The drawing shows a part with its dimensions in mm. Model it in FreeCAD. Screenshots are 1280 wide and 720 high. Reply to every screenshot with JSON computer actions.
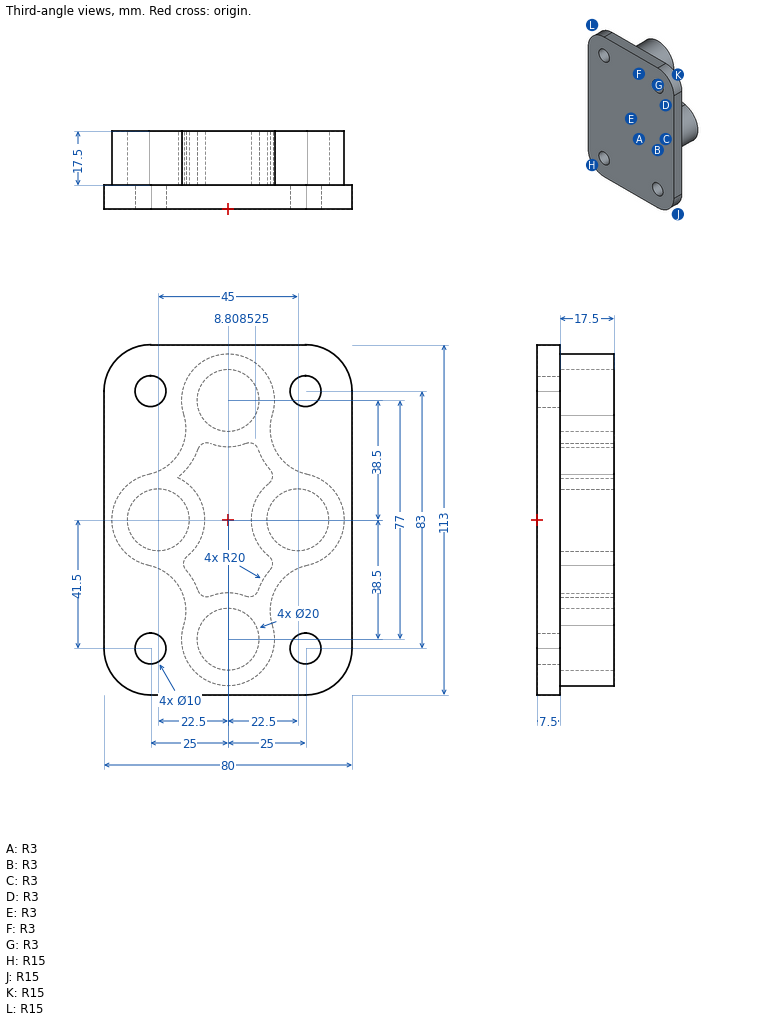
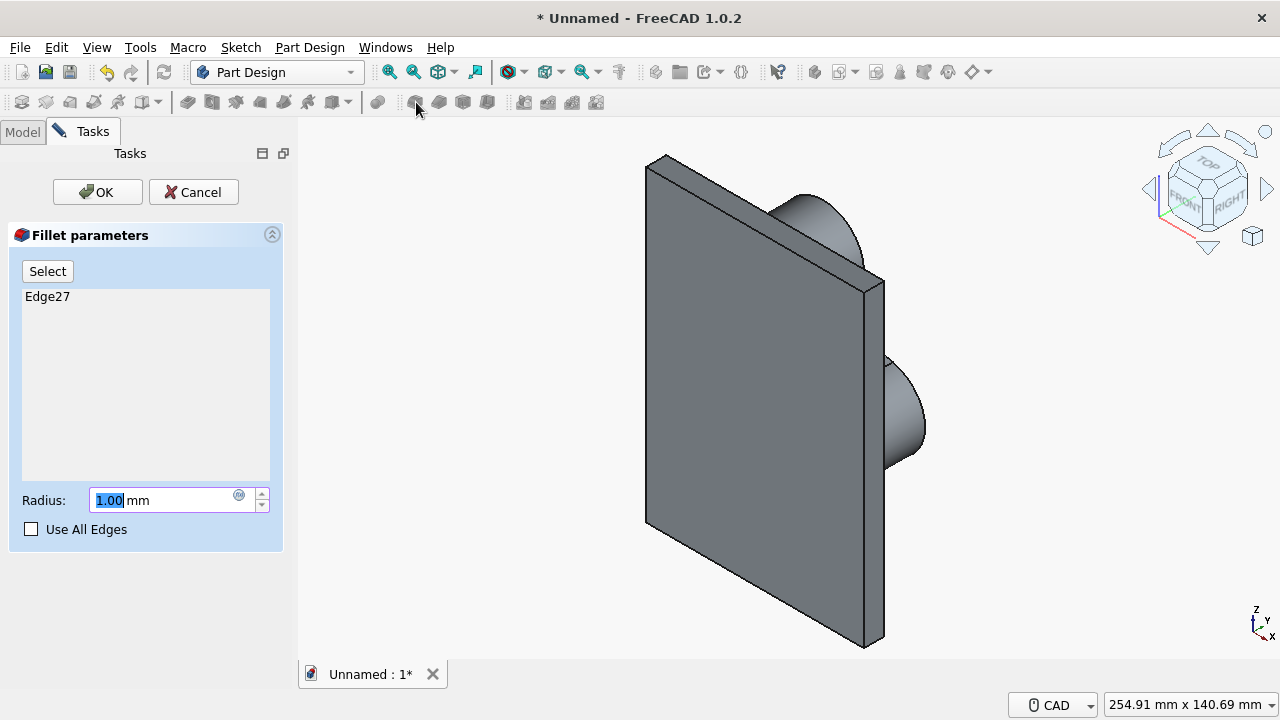
{"action": "type", "text": "3"}
{"action": "key", "text": "Tab"}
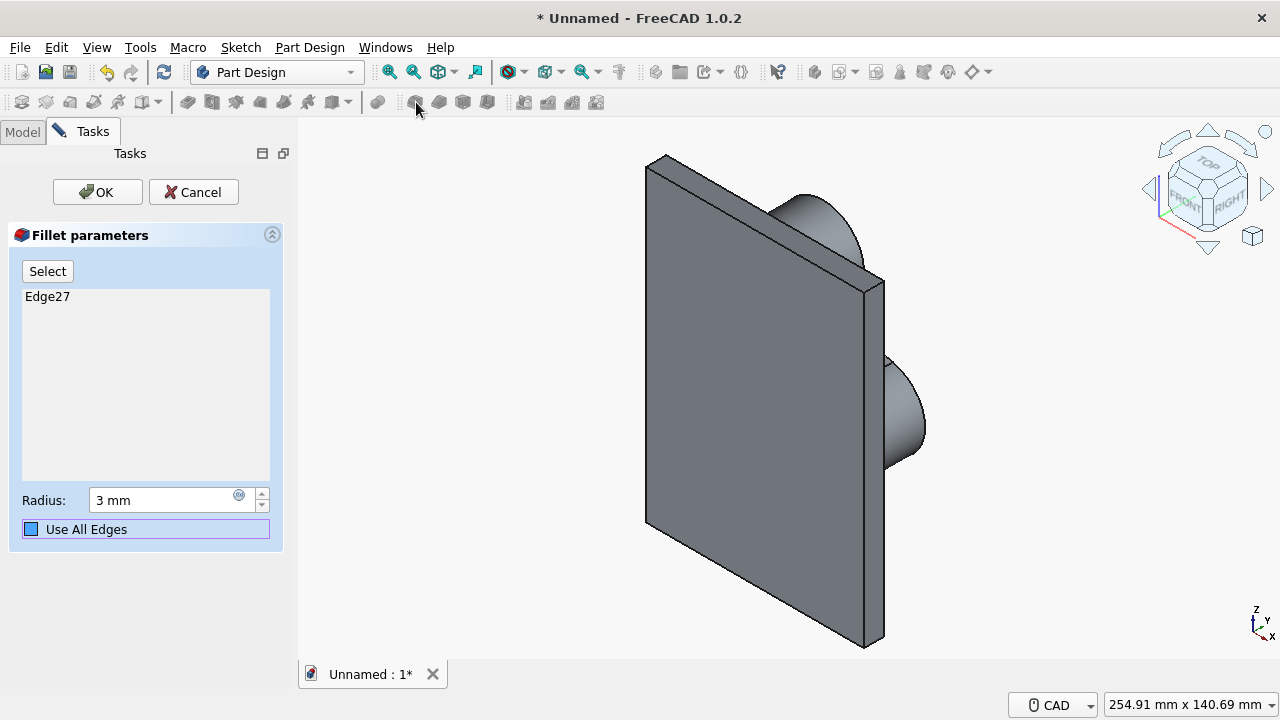
{"action": "left_click", "coordinate": [98, 192]}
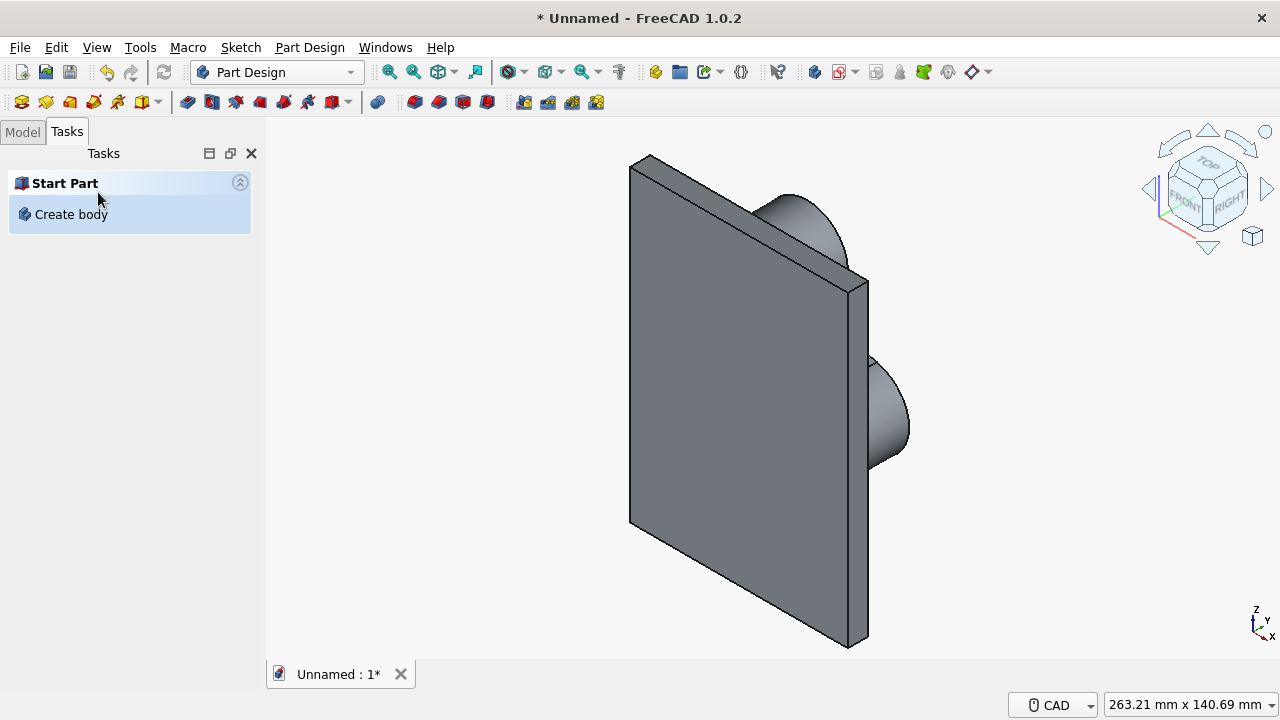
{"action": "key", "text": "2"}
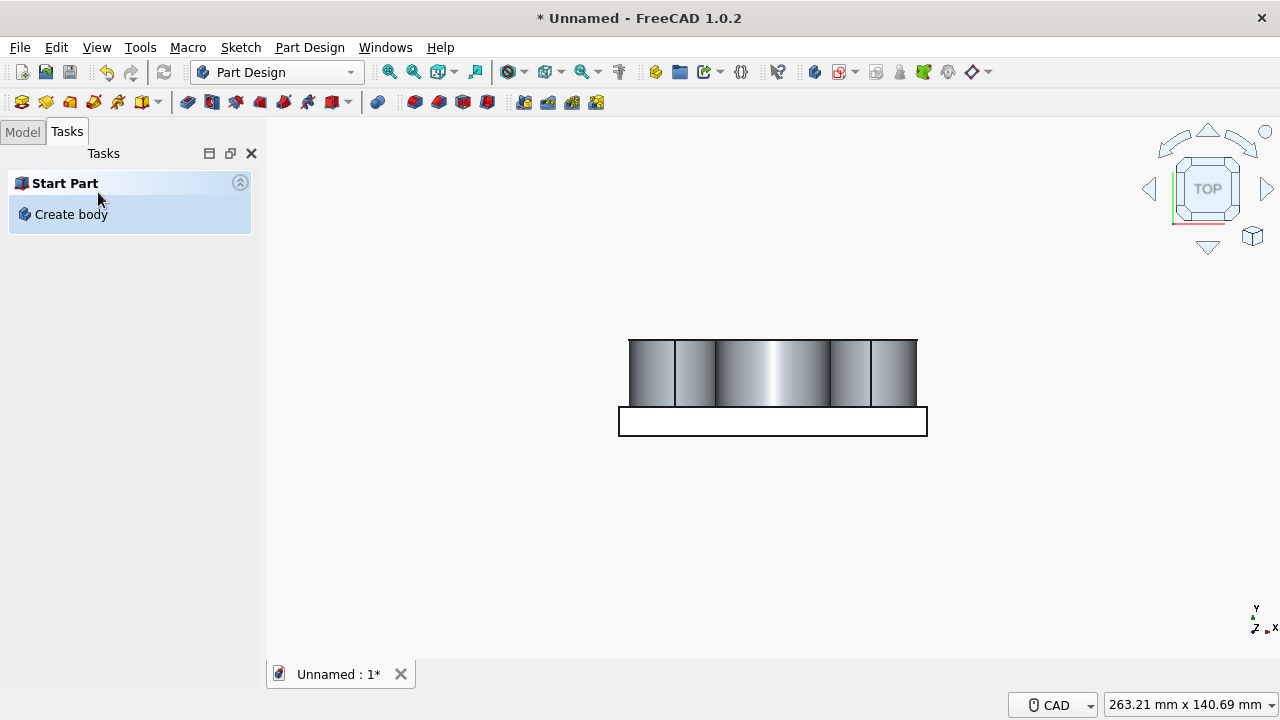
{"action": "left_click", "coordinate": [390, 72]}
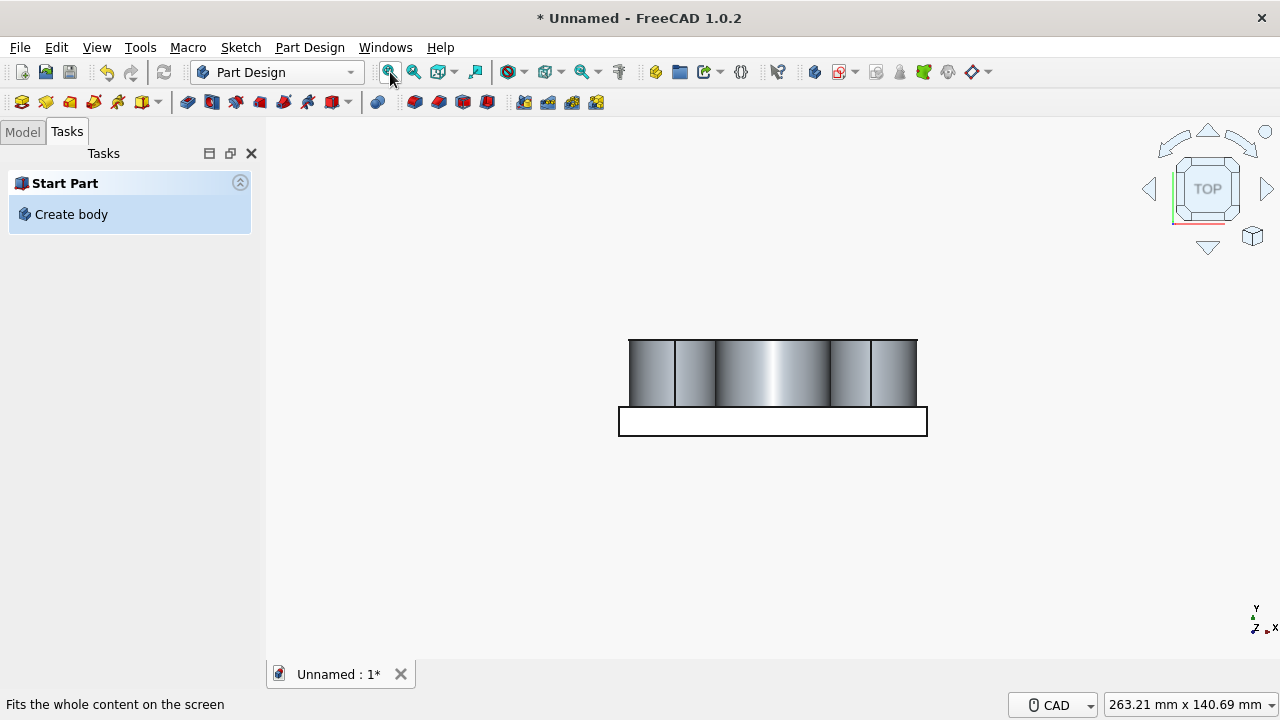
{"action": "key", "text": "0"}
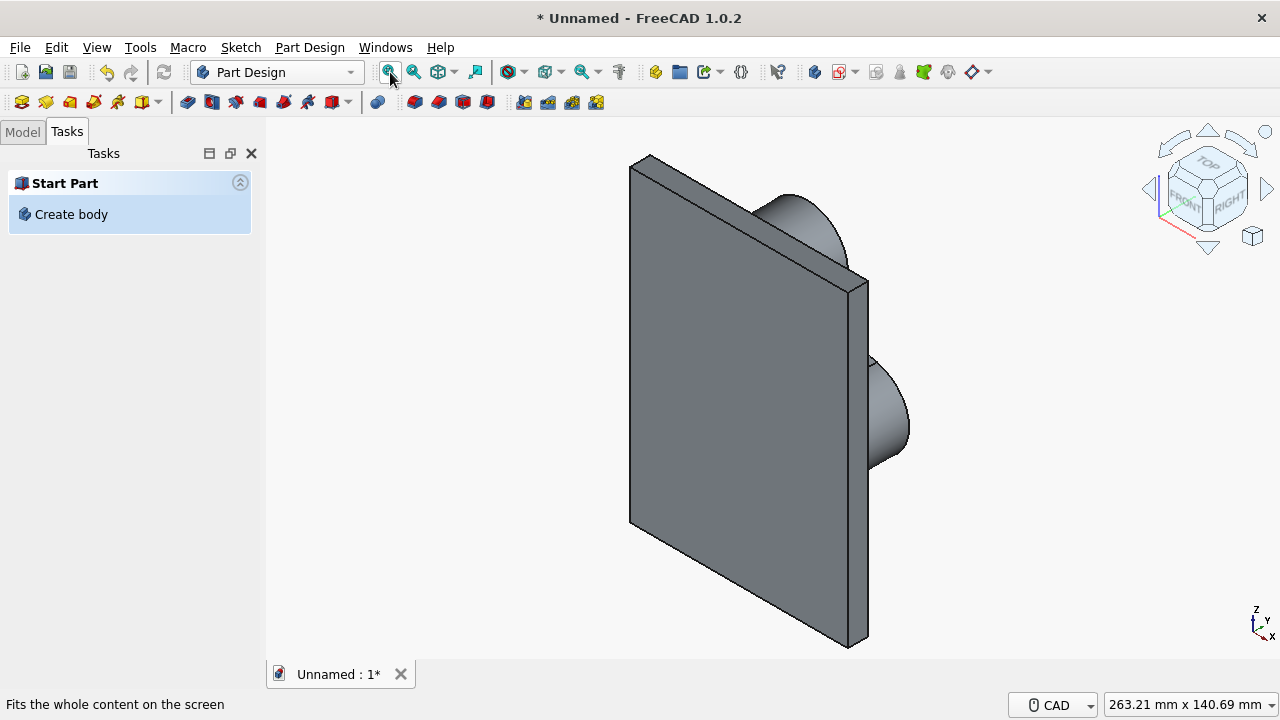
{"action": "key", "text": "1"}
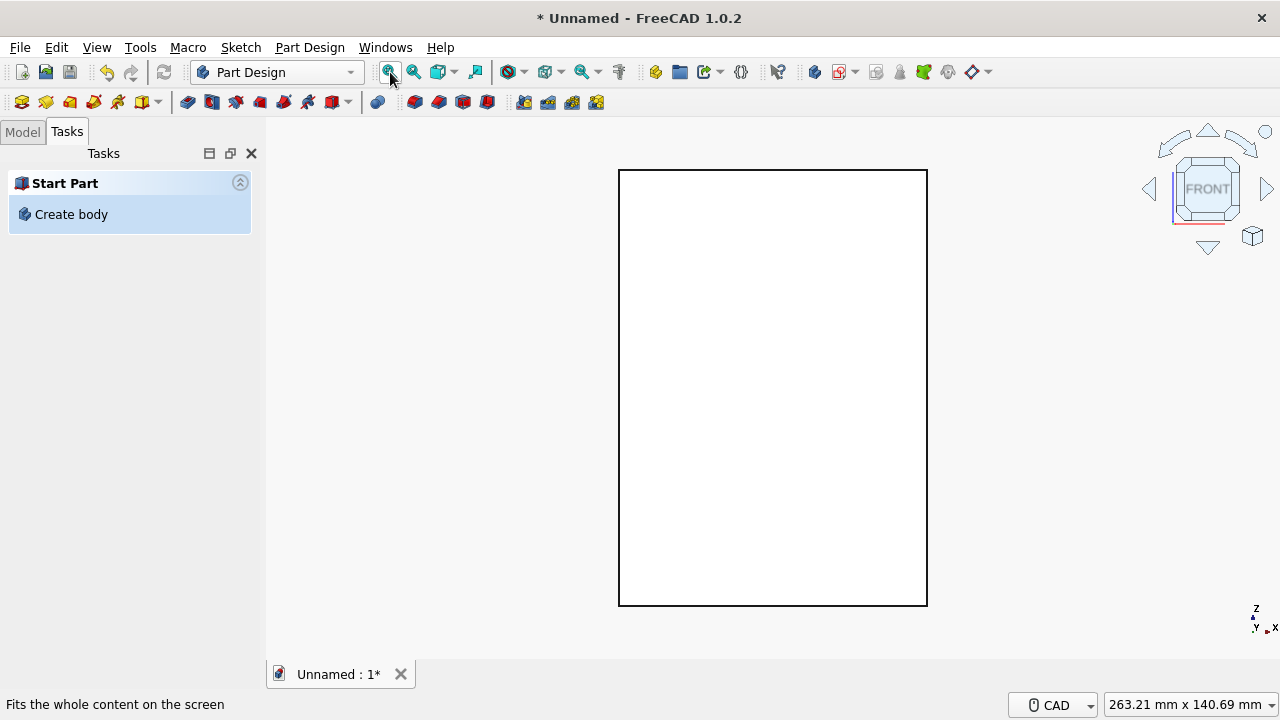
{"action": "key", "text": "3"}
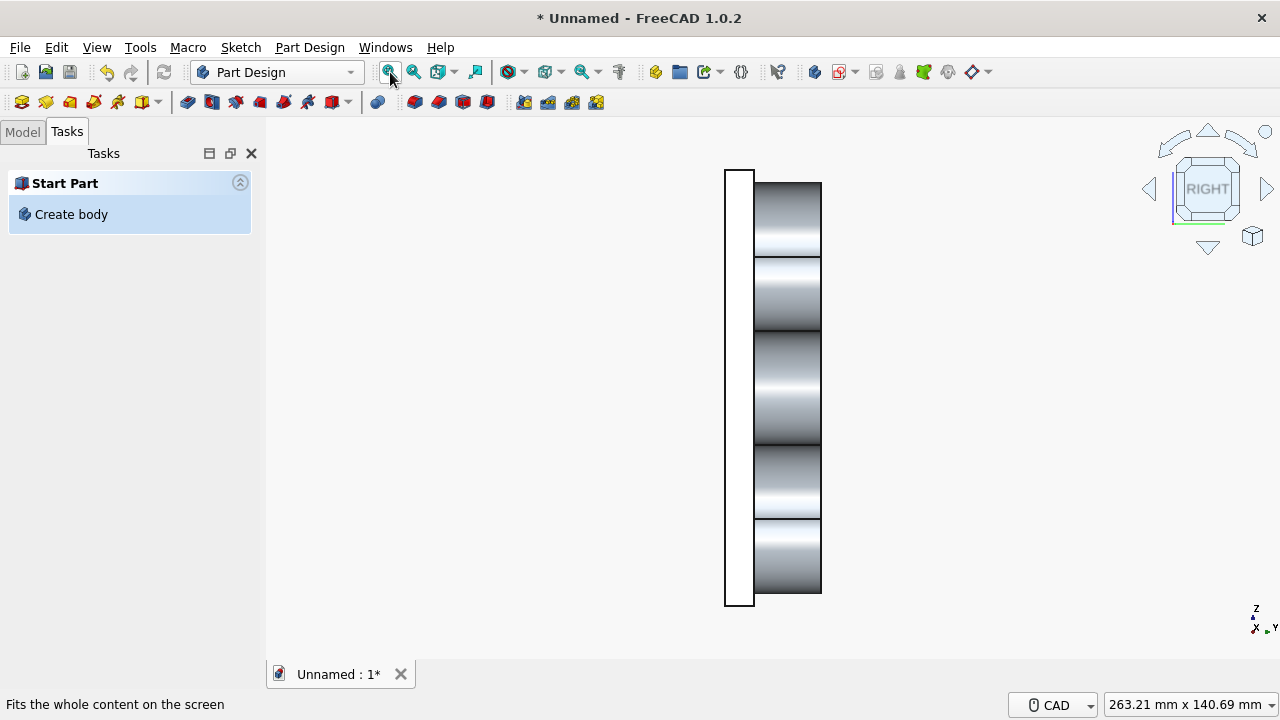
{"action": "key", "text": "5"}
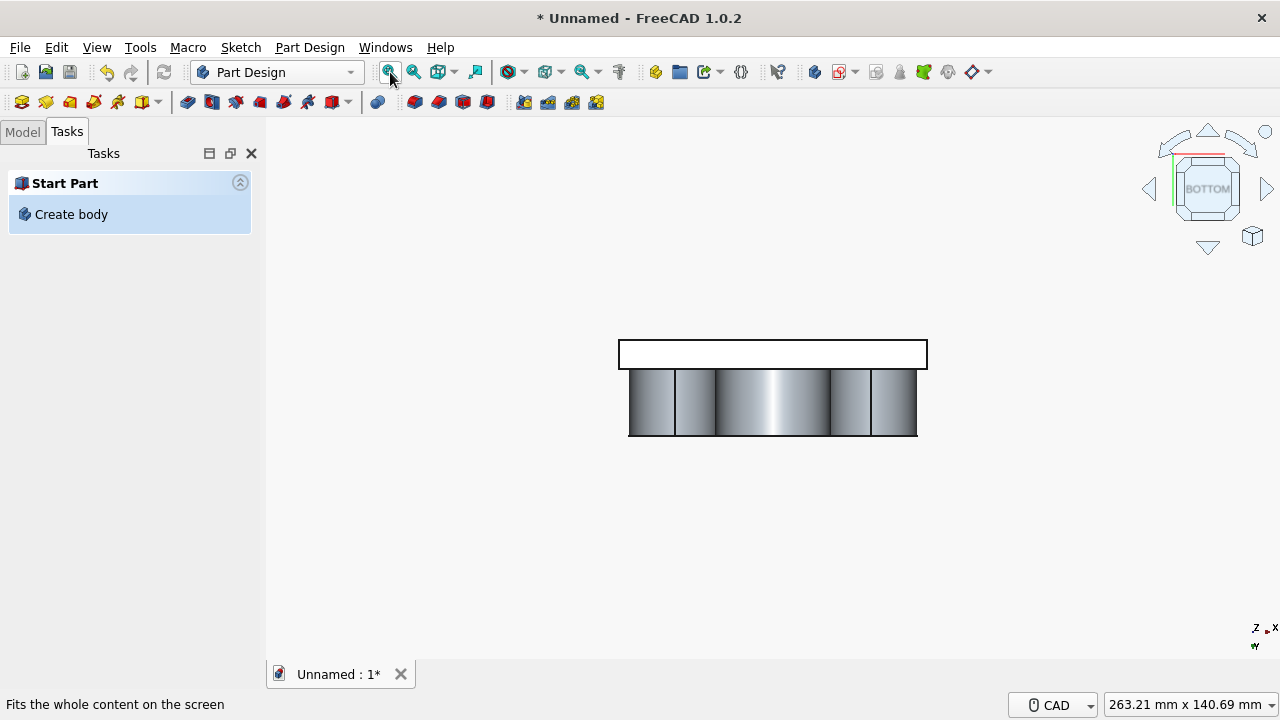
{"action": "key", "text": "v f"}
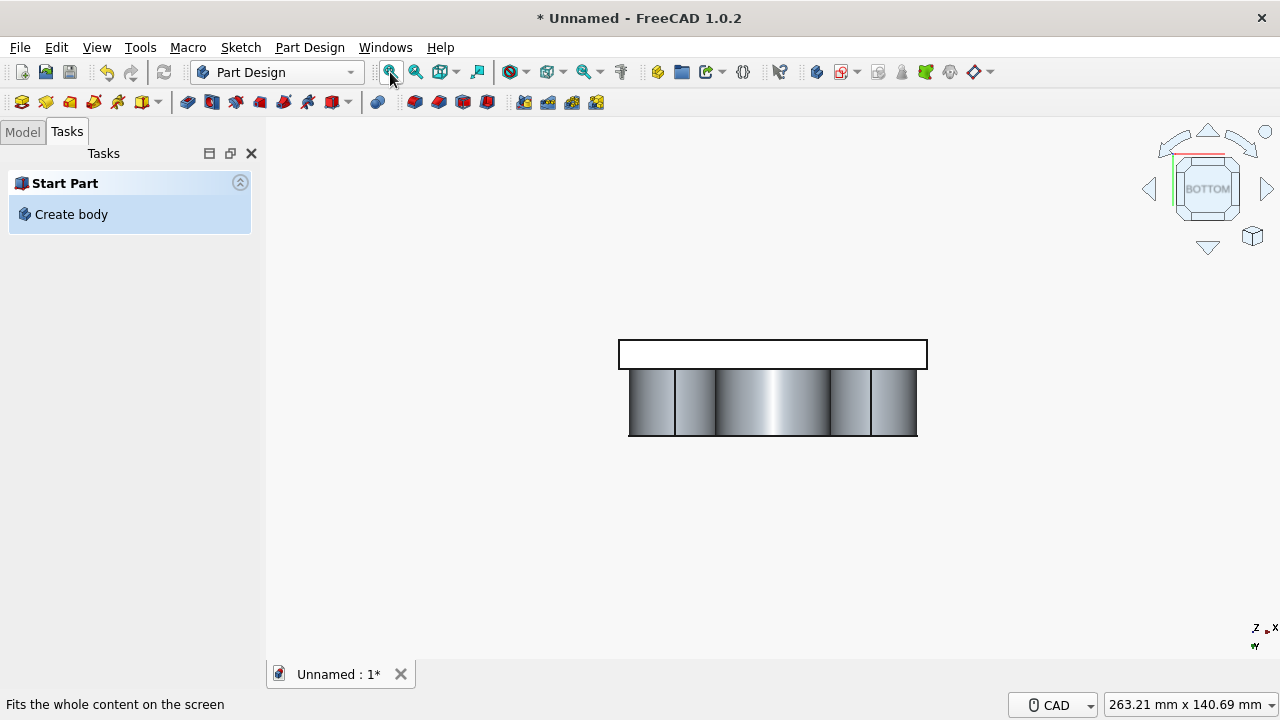
{"action": "key", "text": "4"}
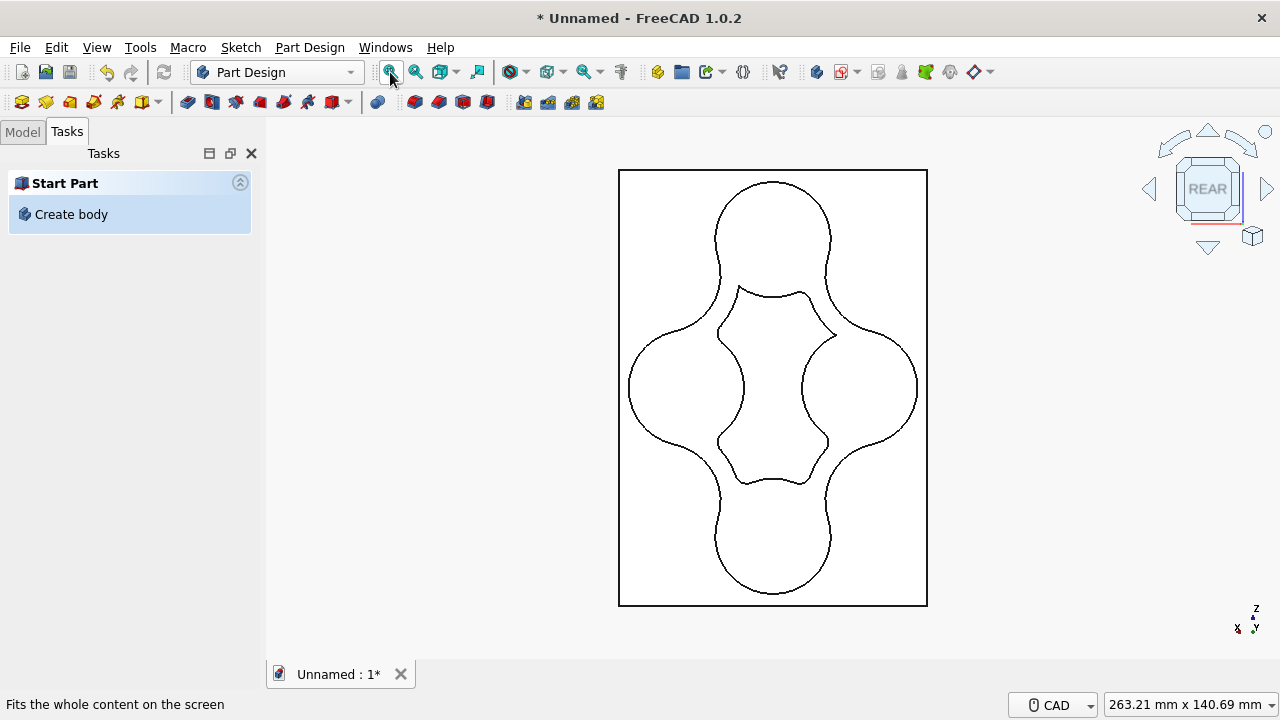
{"action": "key", "text": "6"}